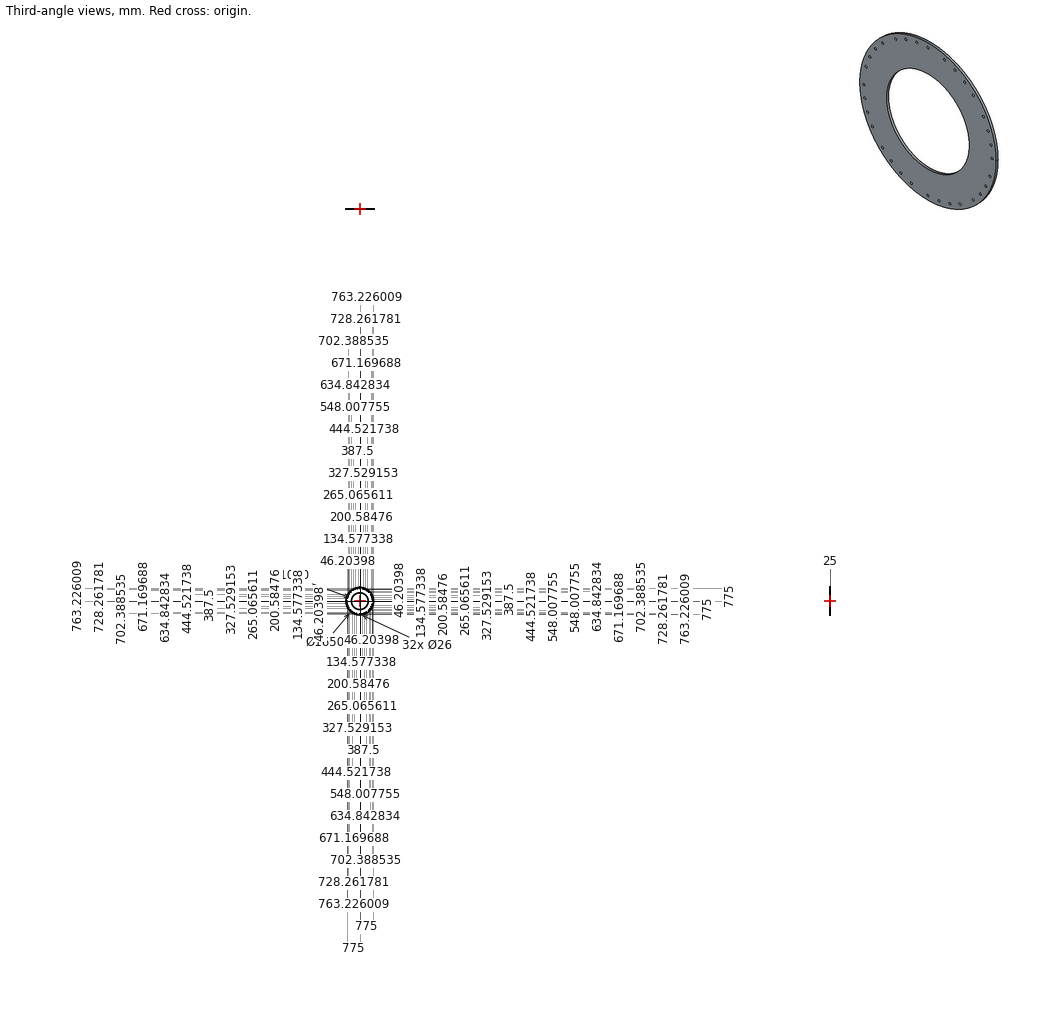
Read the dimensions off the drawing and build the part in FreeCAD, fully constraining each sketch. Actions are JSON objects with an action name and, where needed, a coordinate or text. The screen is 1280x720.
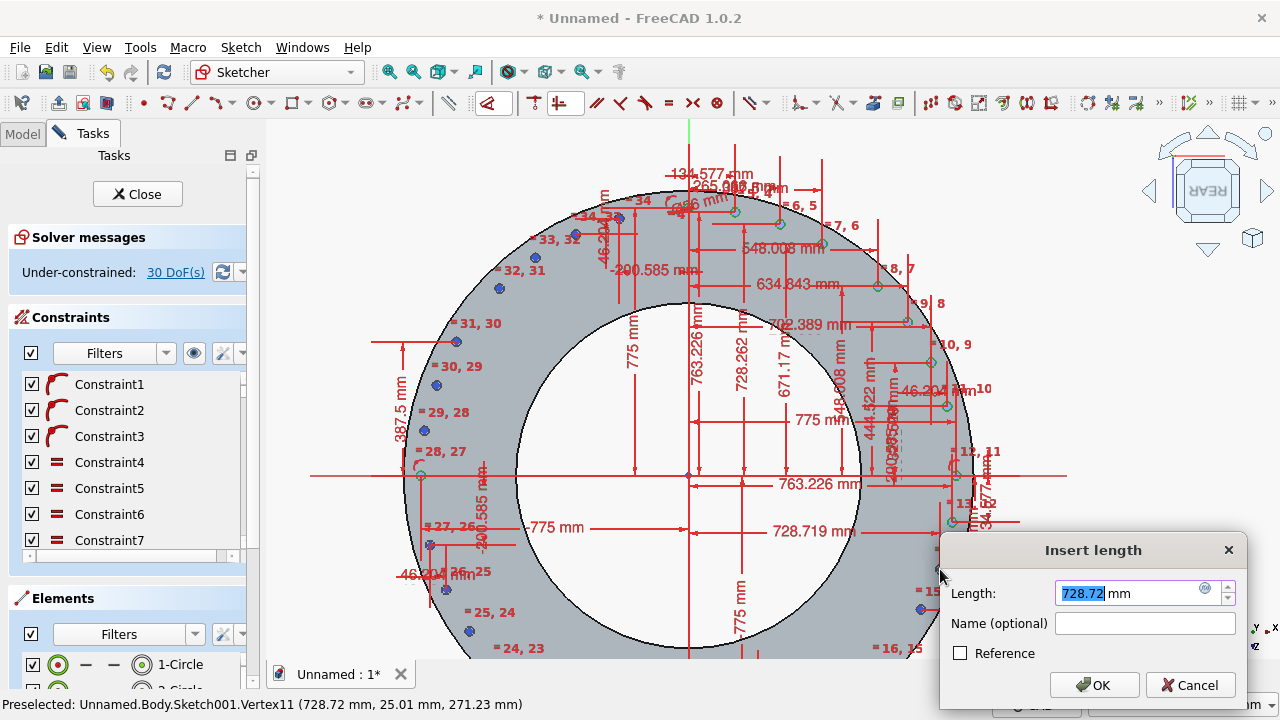
{"action": "type", "text": "728.261781"}
{"action": "key", "text": "Return"}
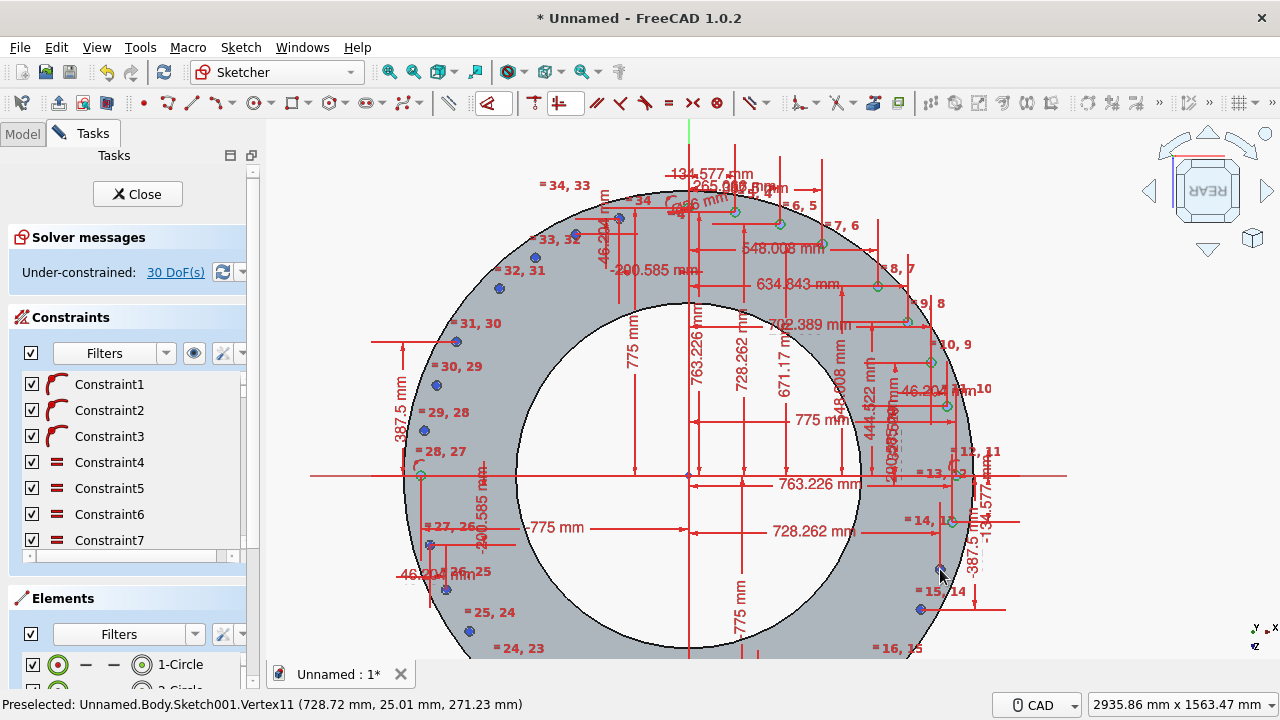
{"action": "left_click", "coordinate": [940, 569]}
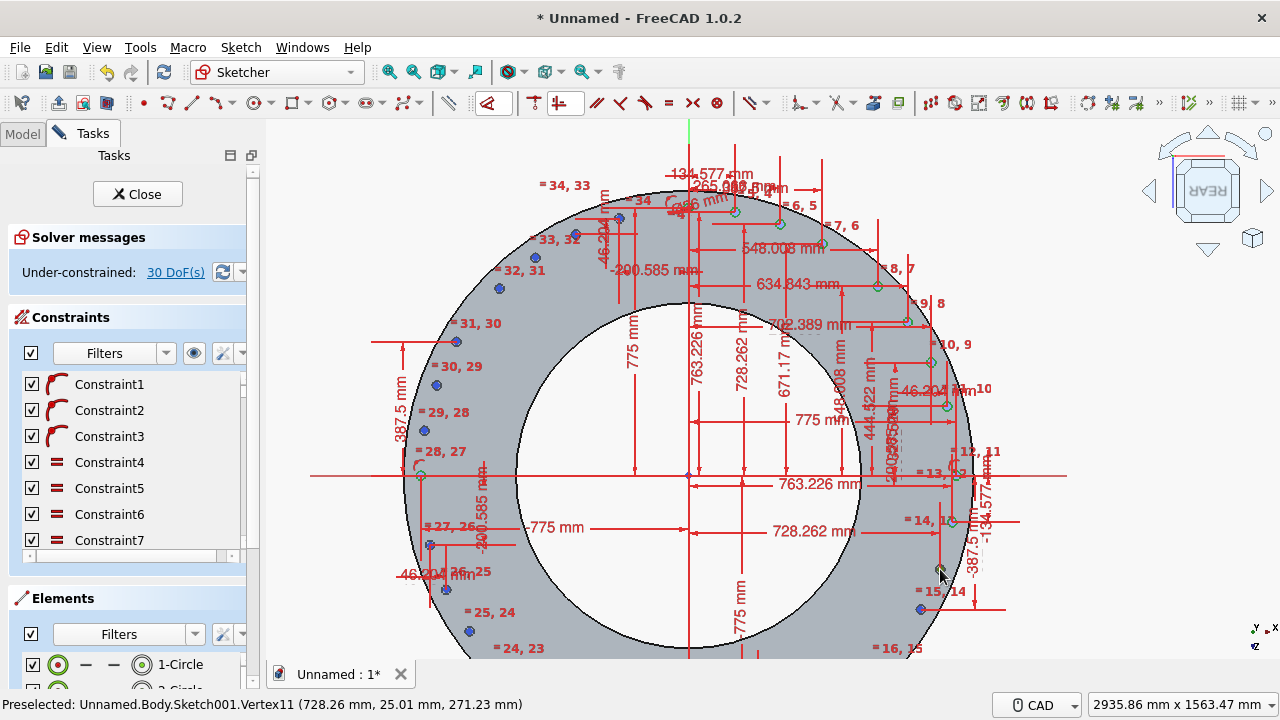
{"action": "key", "text": "i"}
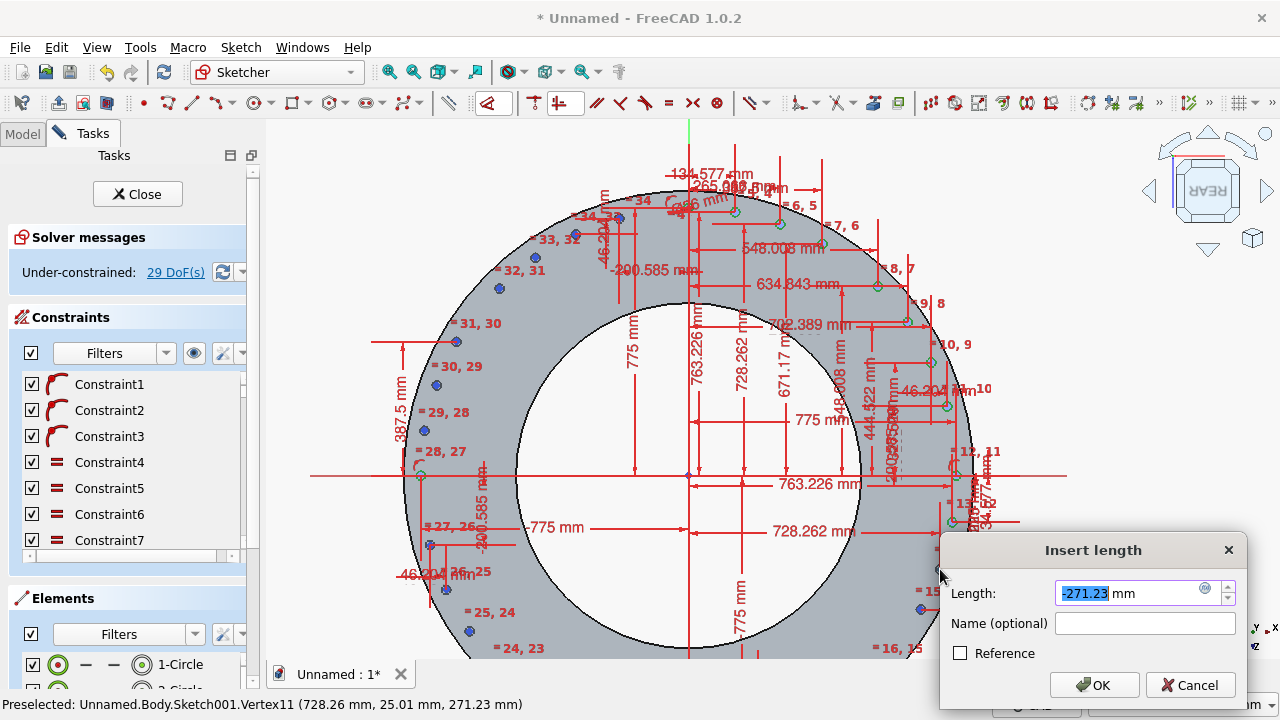
{"action": "type", "text": "-265.065611"}
{"action": "key", "text": "Return"}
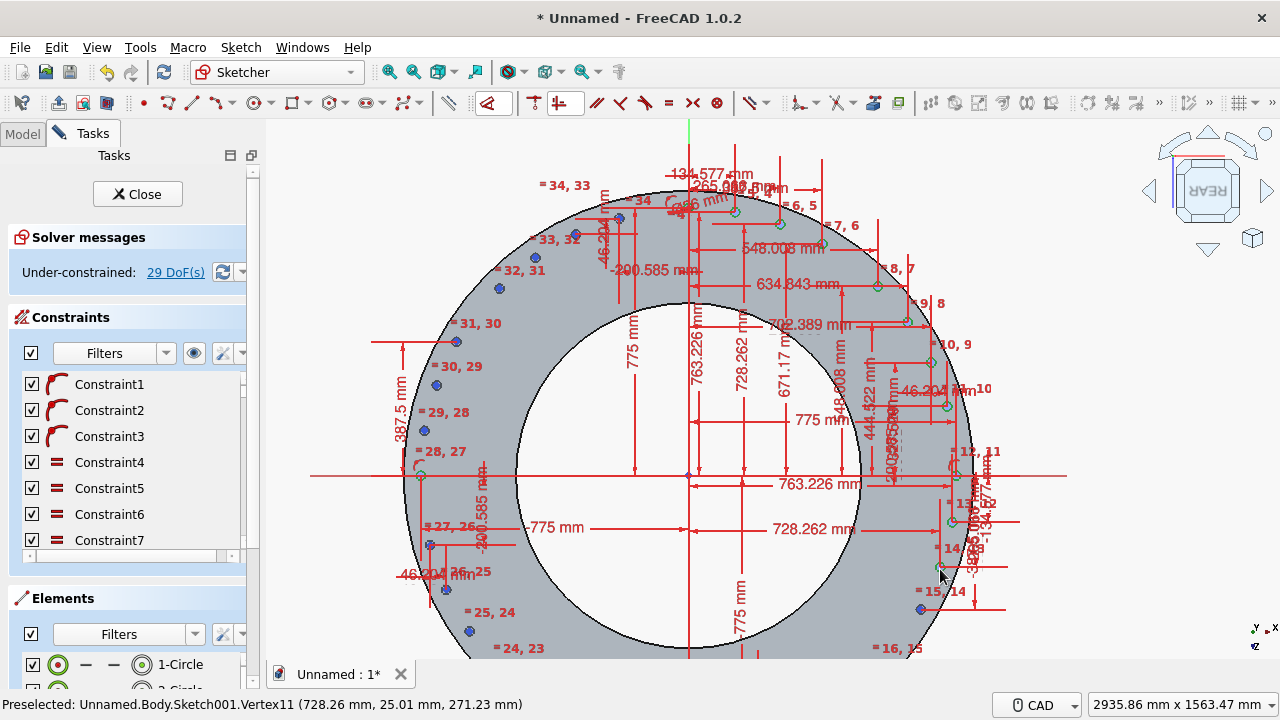
{"action": "left_click", "coordinate": [921, 610]}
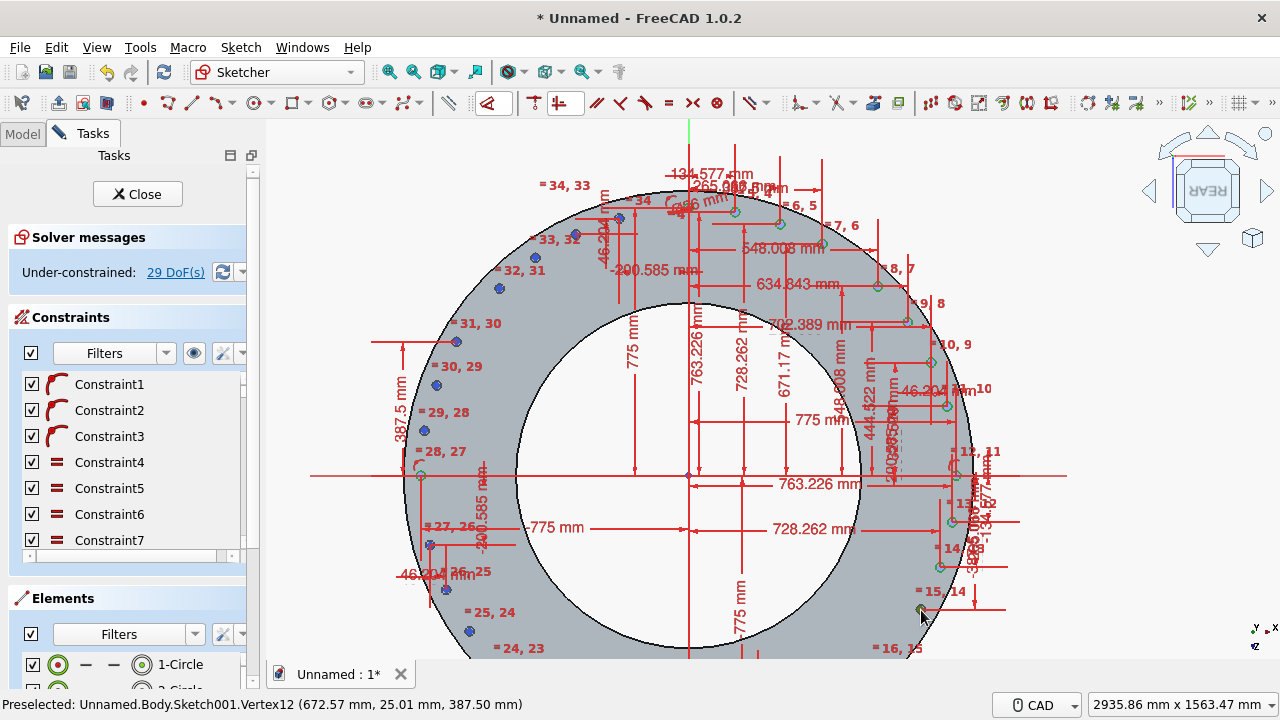
{"action": "key", "text": "l"}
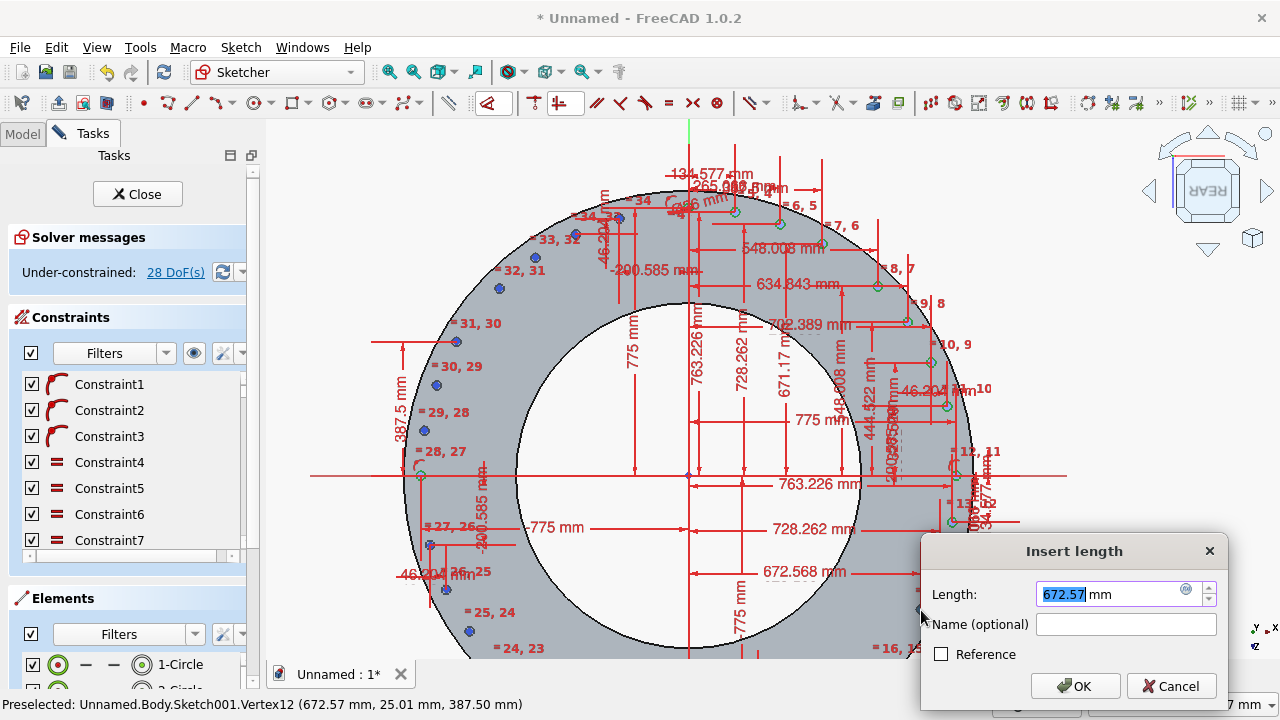
{"action": "type", "text": "671.169688"}
{"action": "key", "text": "Return"}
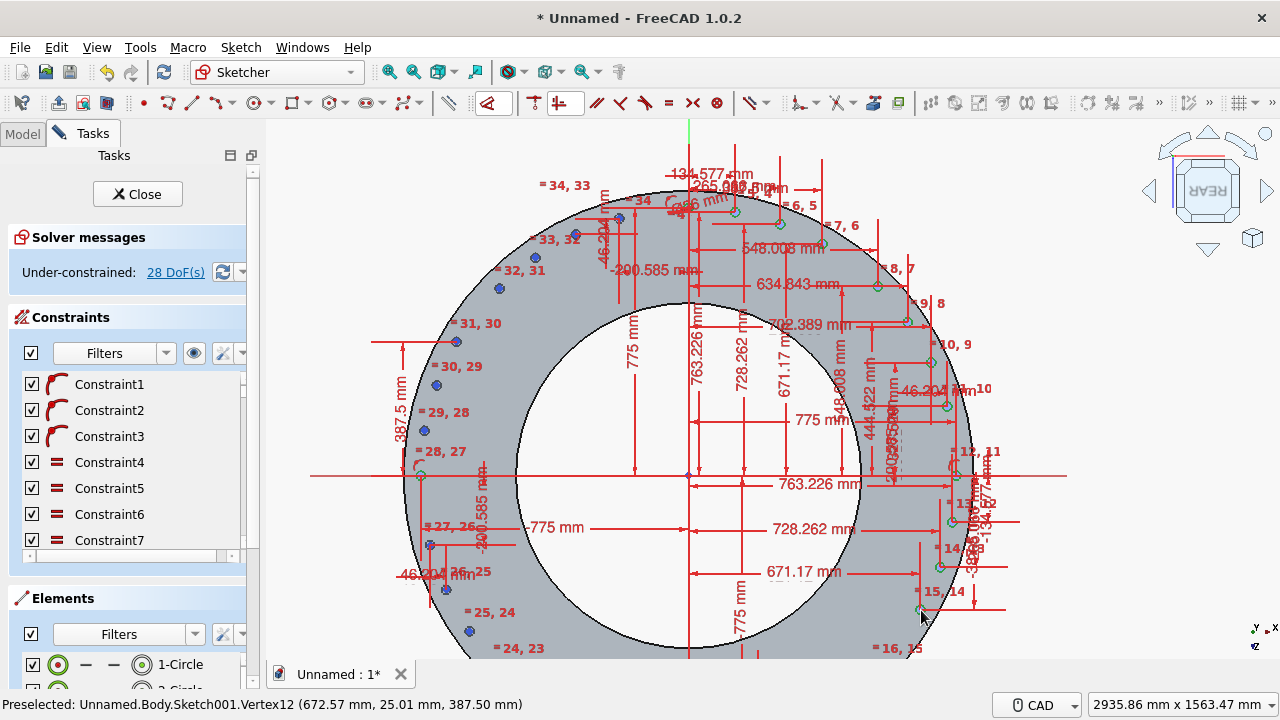
{"action": "scroll", "coordinate": [737, 213], "scroll_direction": "down", "scroll_amount": 2}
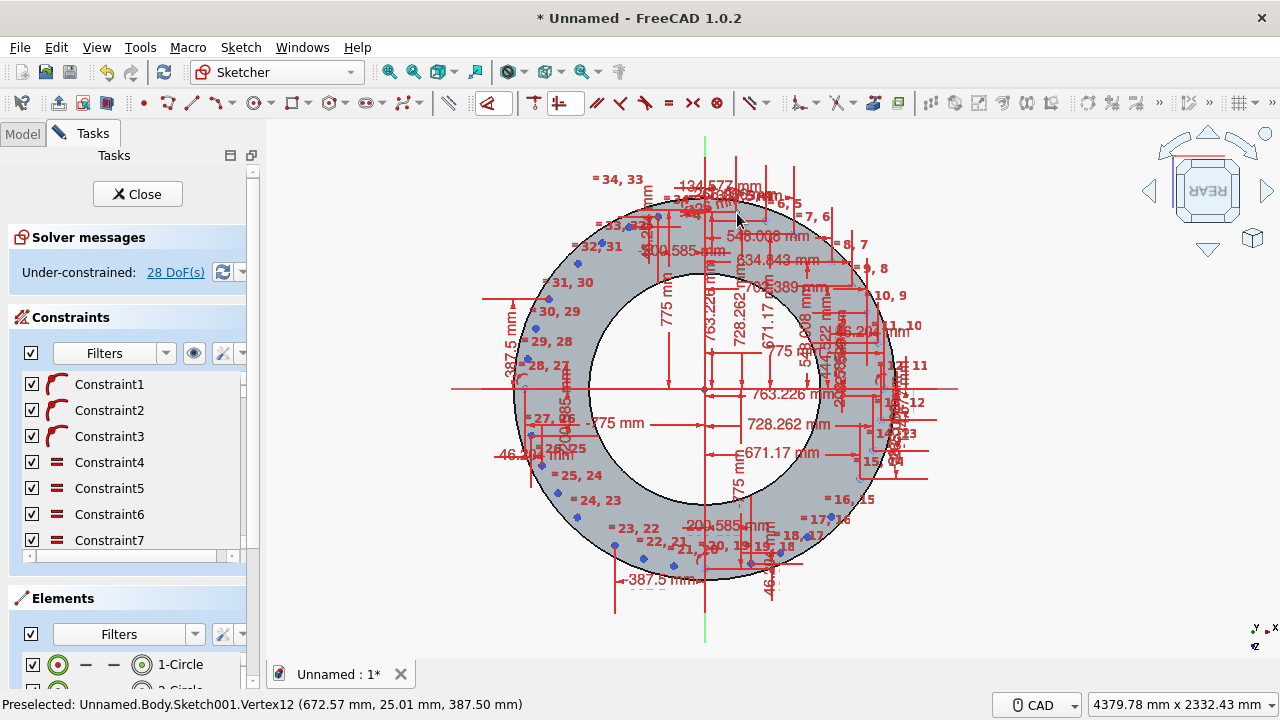
{"action": "left_click", "coordinate": [831, 517]}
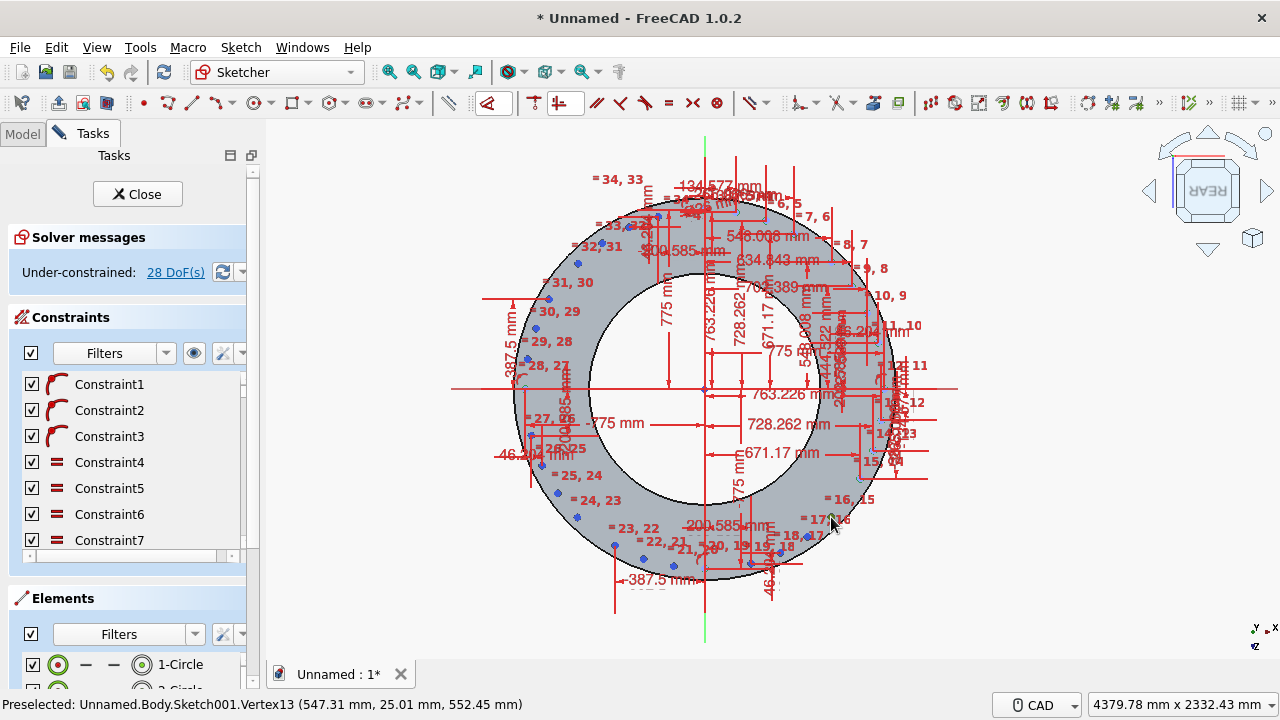
{"action": "key", "text": "l"}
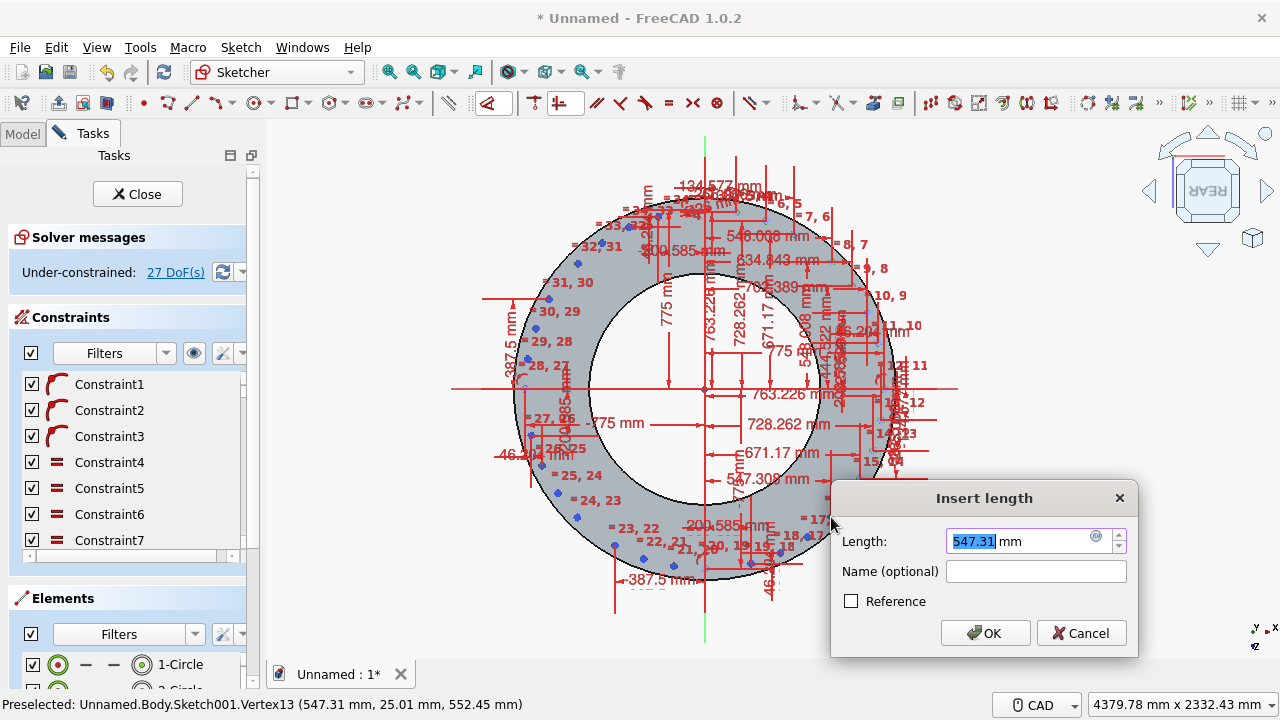
{"action": "type", "text": "548.007755"}
{"action": "key", "text": "Return"}